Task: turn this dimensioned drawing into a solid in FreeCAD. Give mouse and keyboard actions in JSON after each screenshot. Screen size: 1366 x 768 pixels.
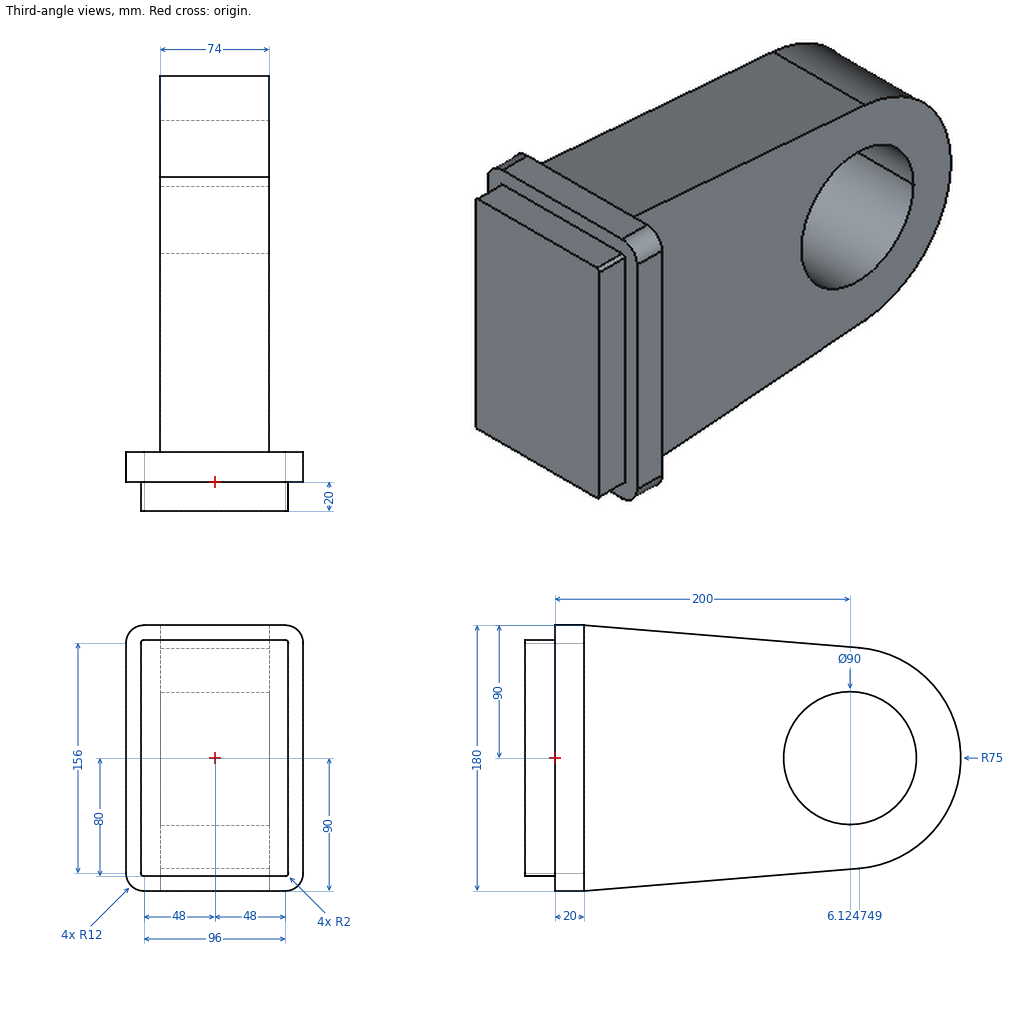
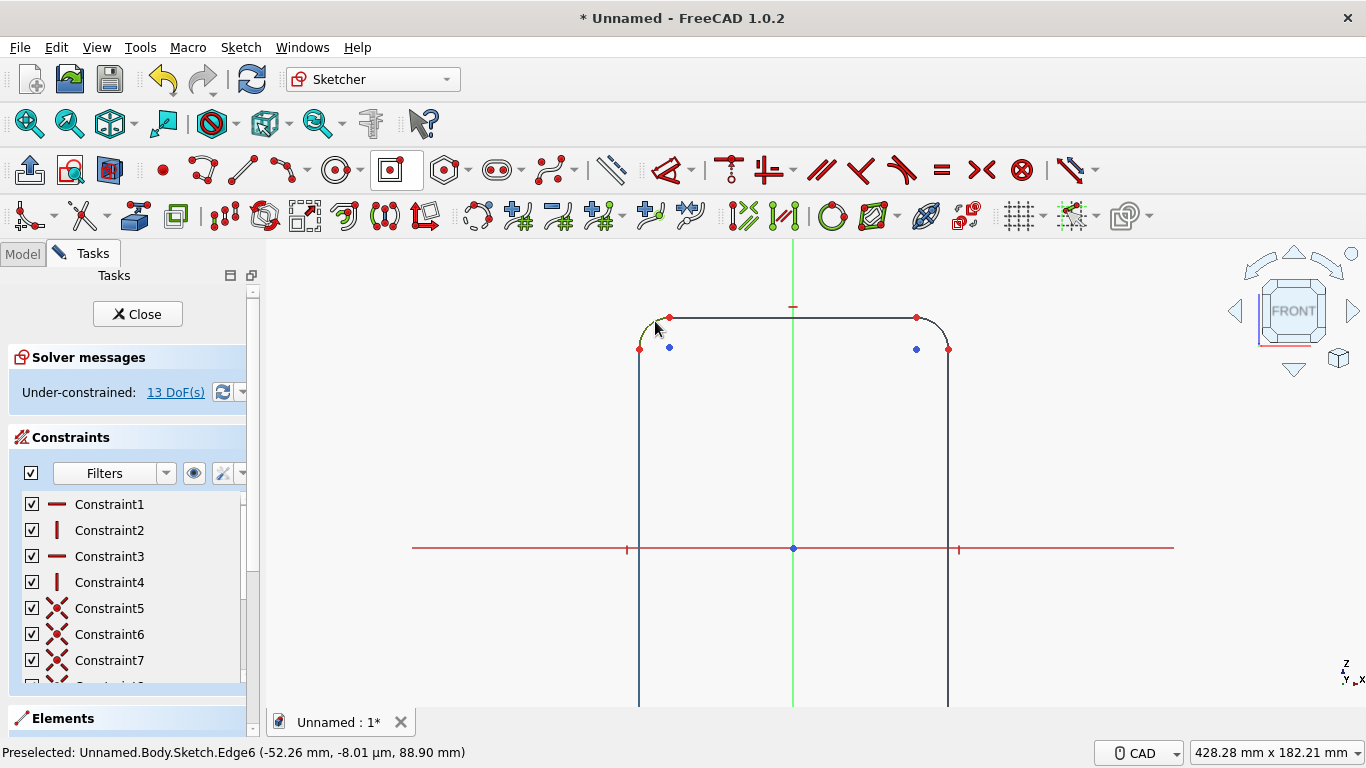
{"action": "key", "text": "t"}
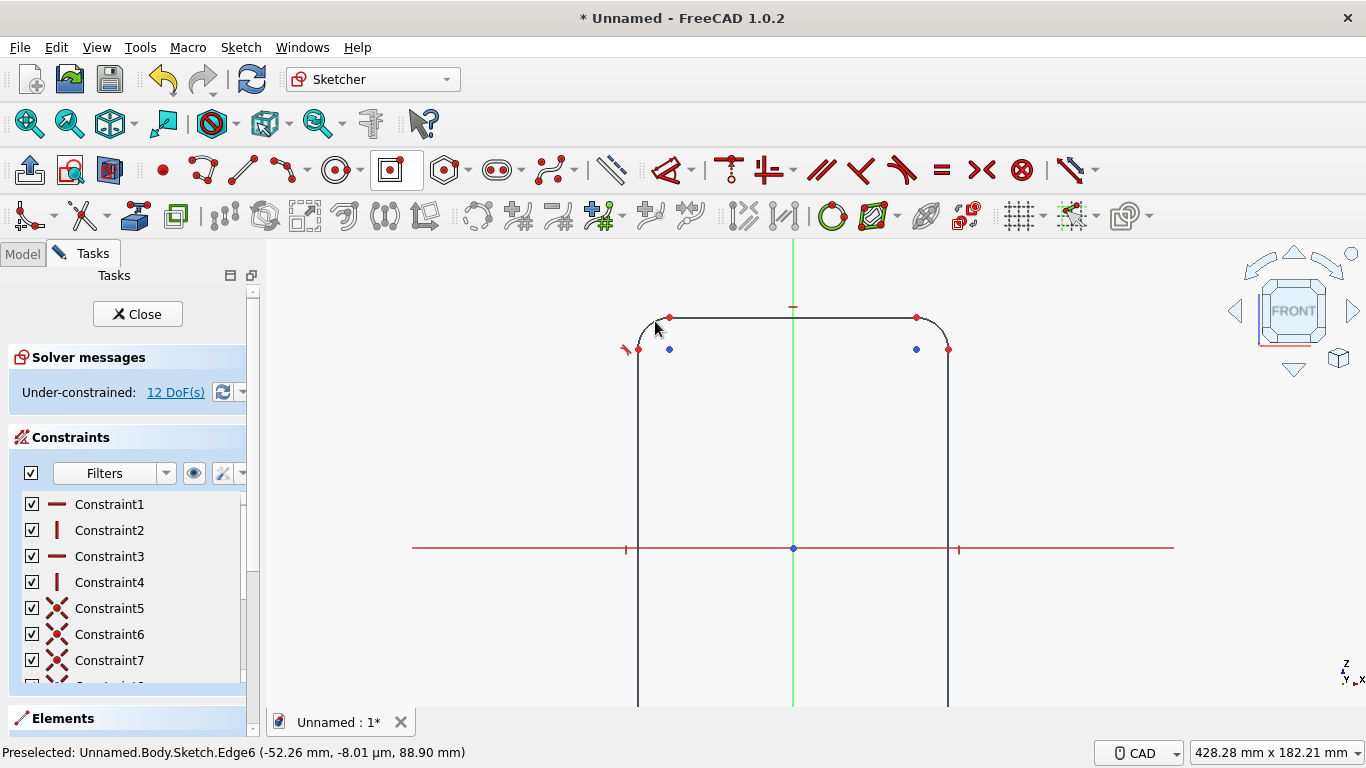
{"action": "left_click", "coordinate": [744, 318]}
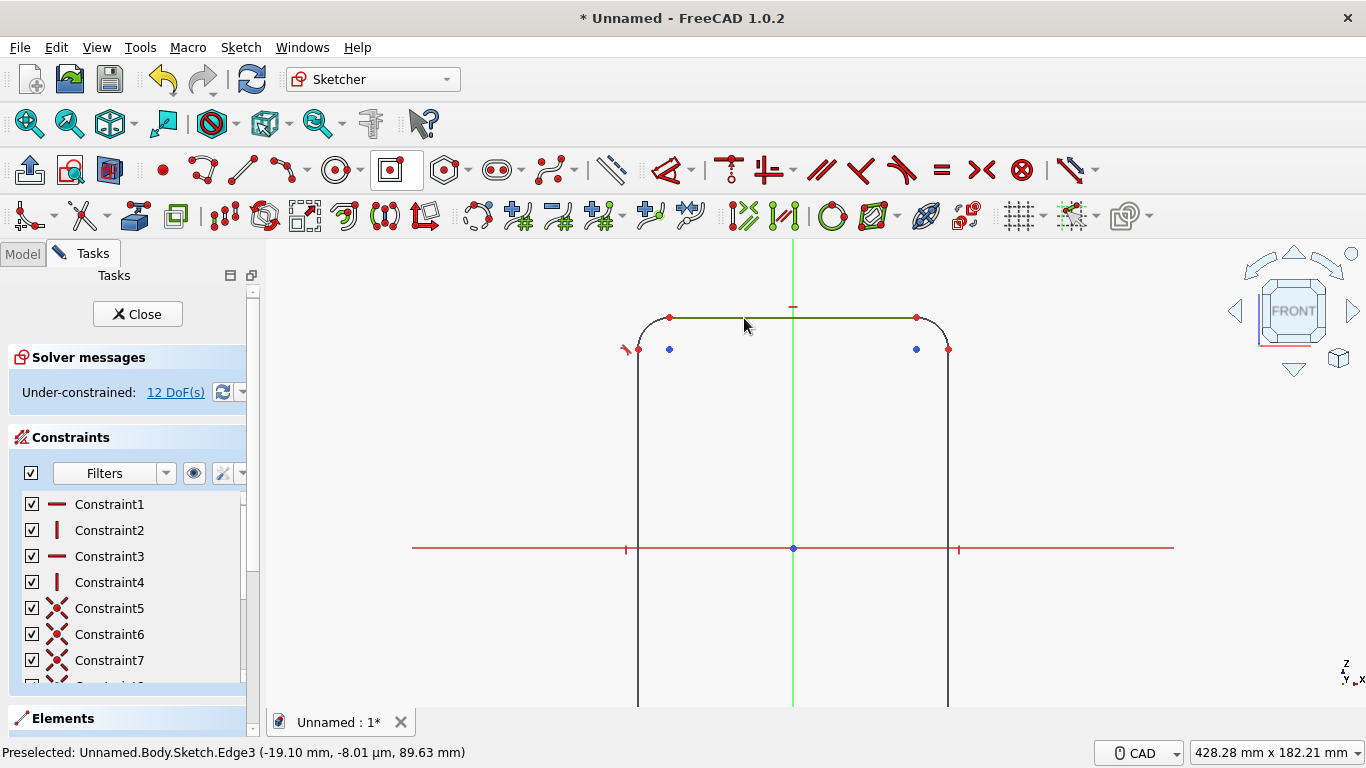
{"action": "left_click", "coordinate": [655, 321]}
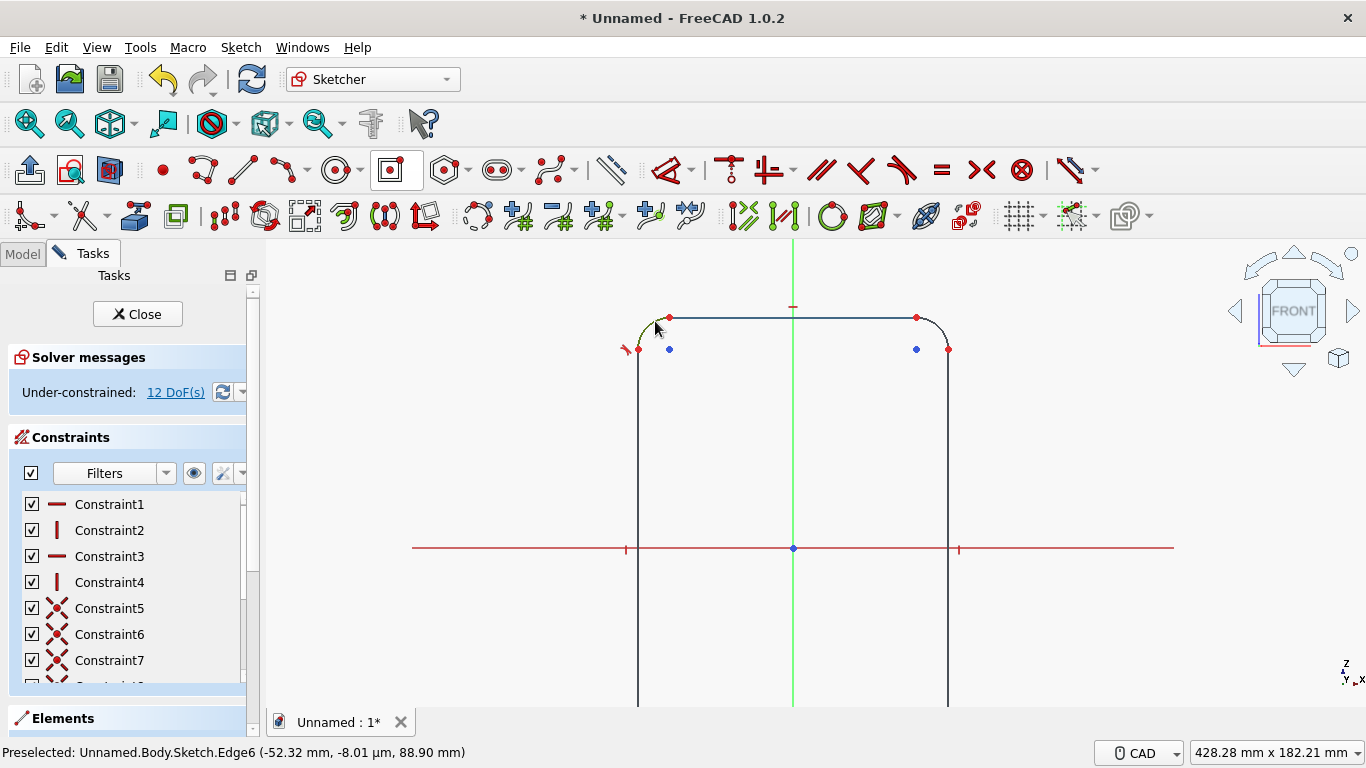
{"action": "left_click", "coordinate": [902, 170]}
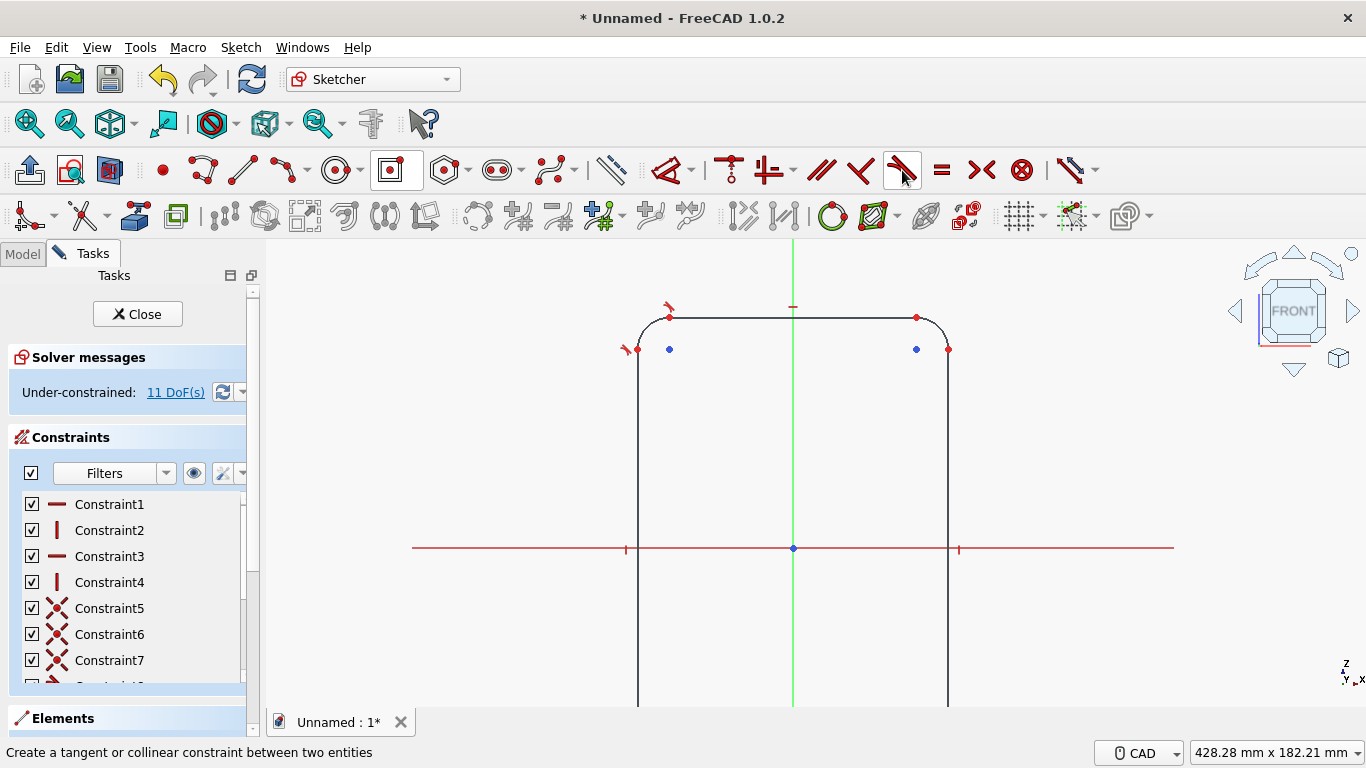
{"action": "left_click", "coordinate": [744, 318]}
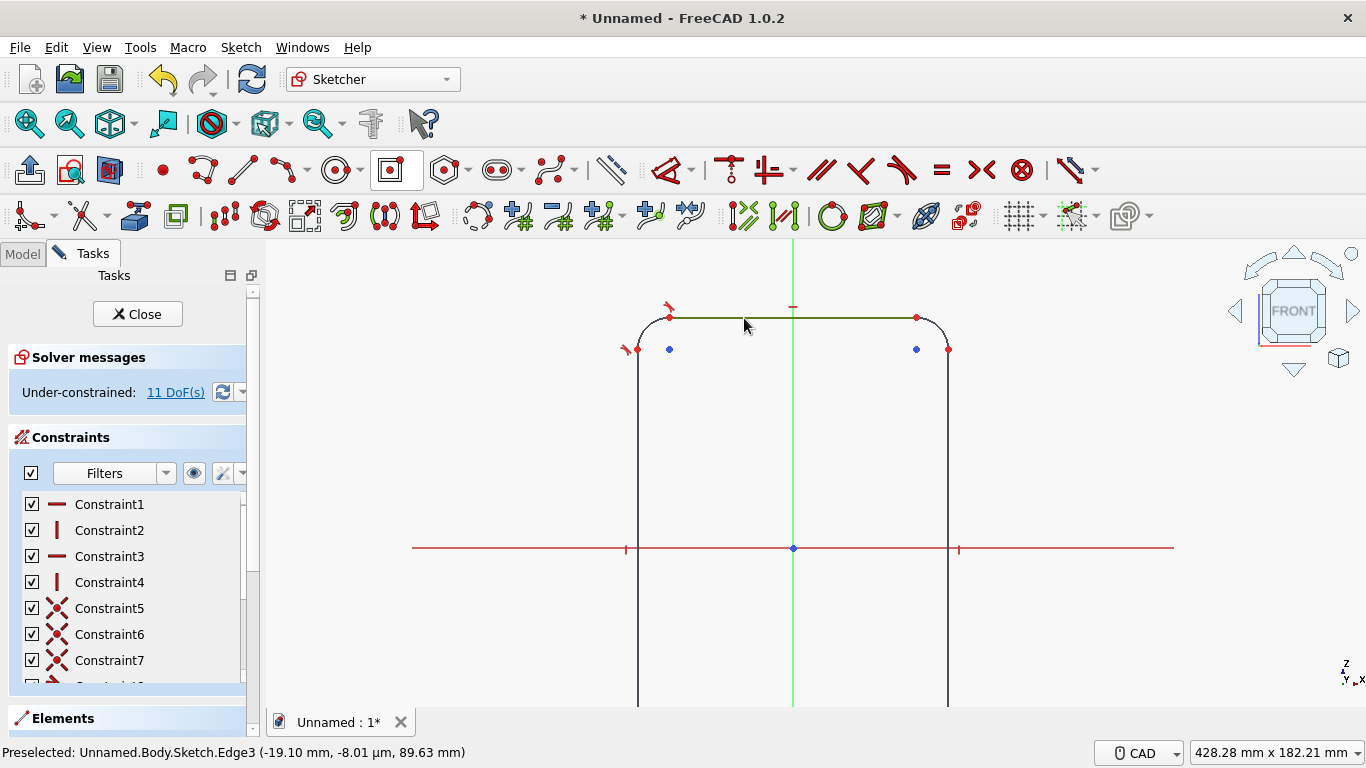
{"action": "left_click", "coordinate": [945, 335]}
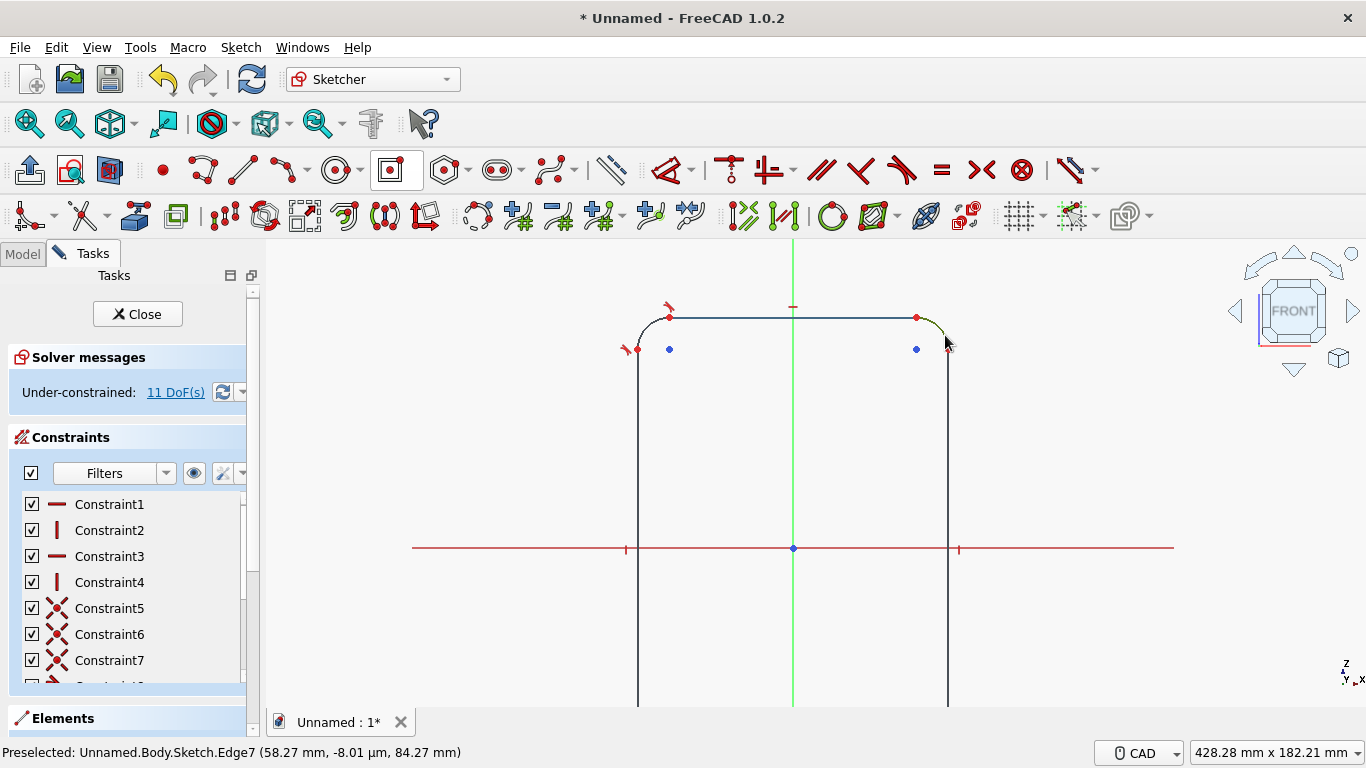
{"action": "key", "text": "t"}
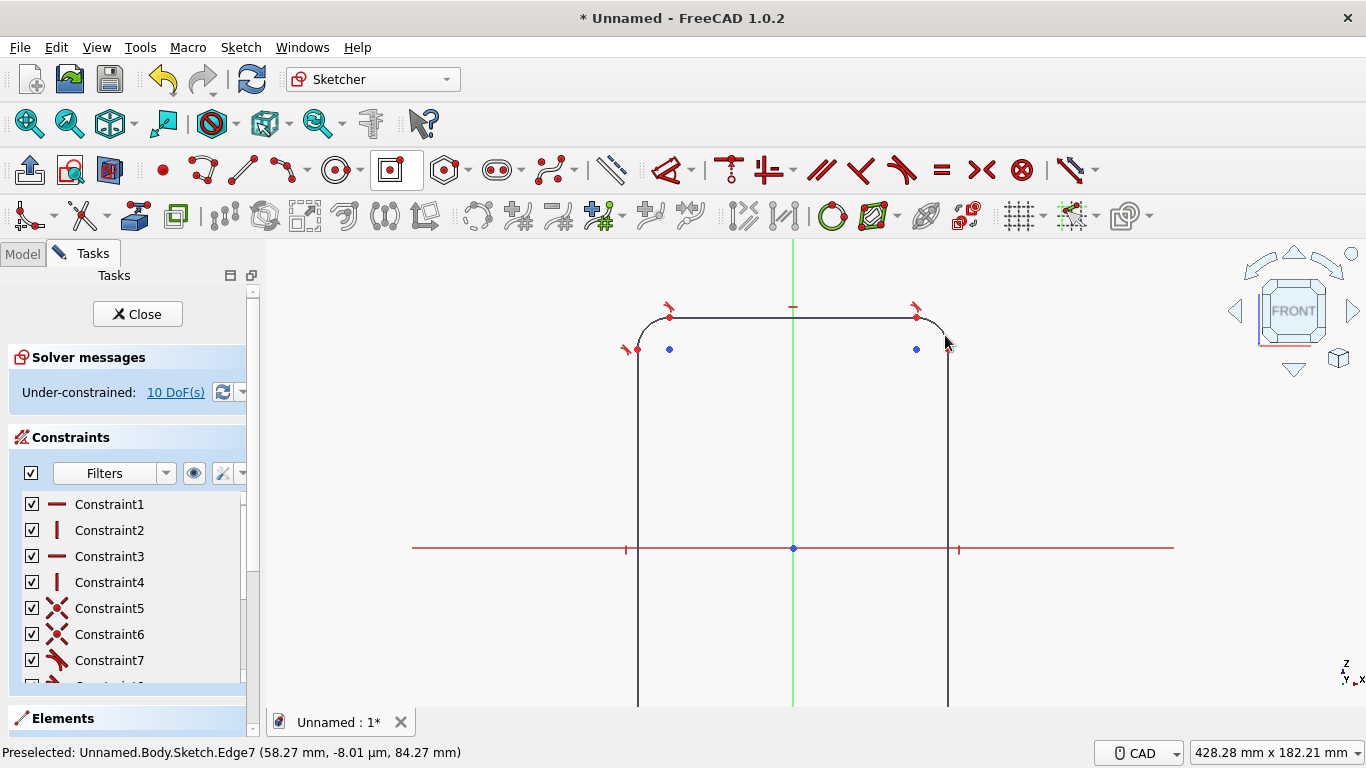
{"action": "left_click", "coordinate": [948, 470]}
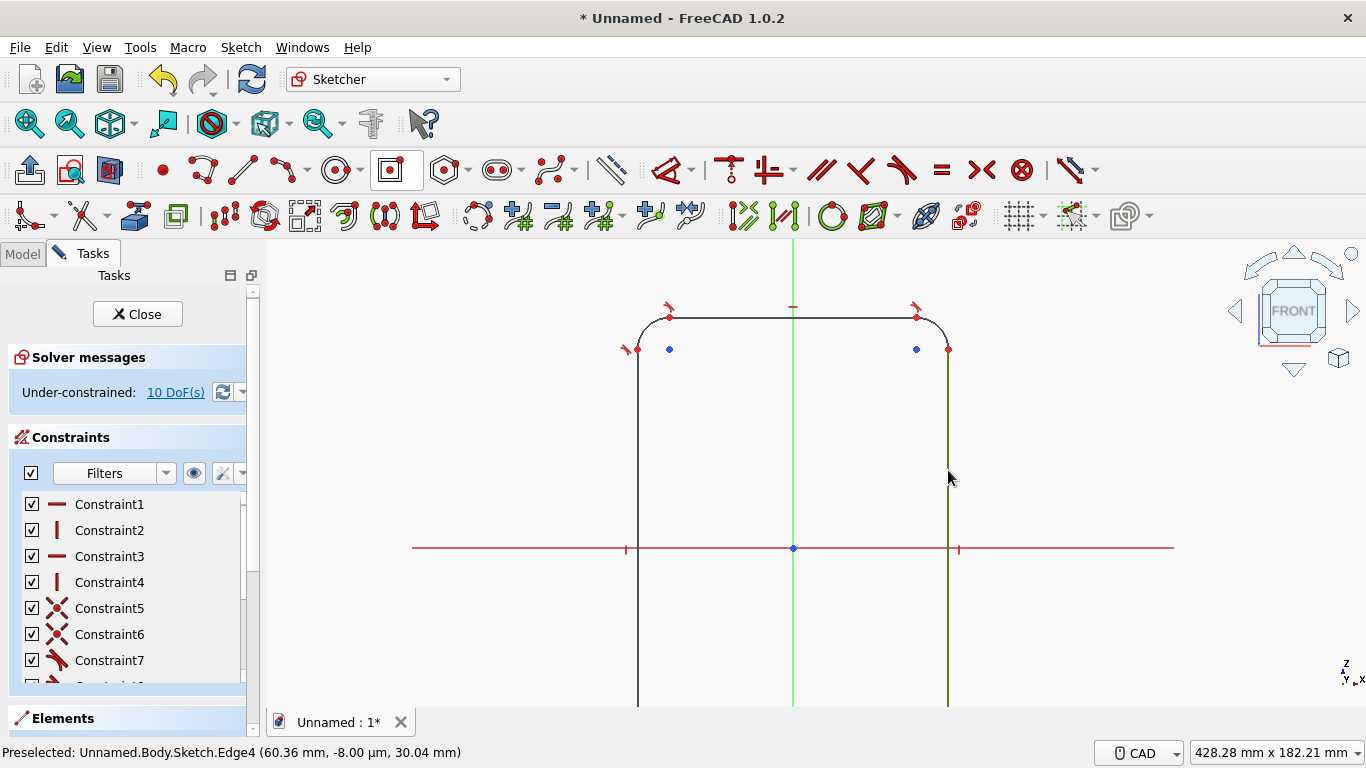
{"action": "left_click", "coordinate": [945, 335]}